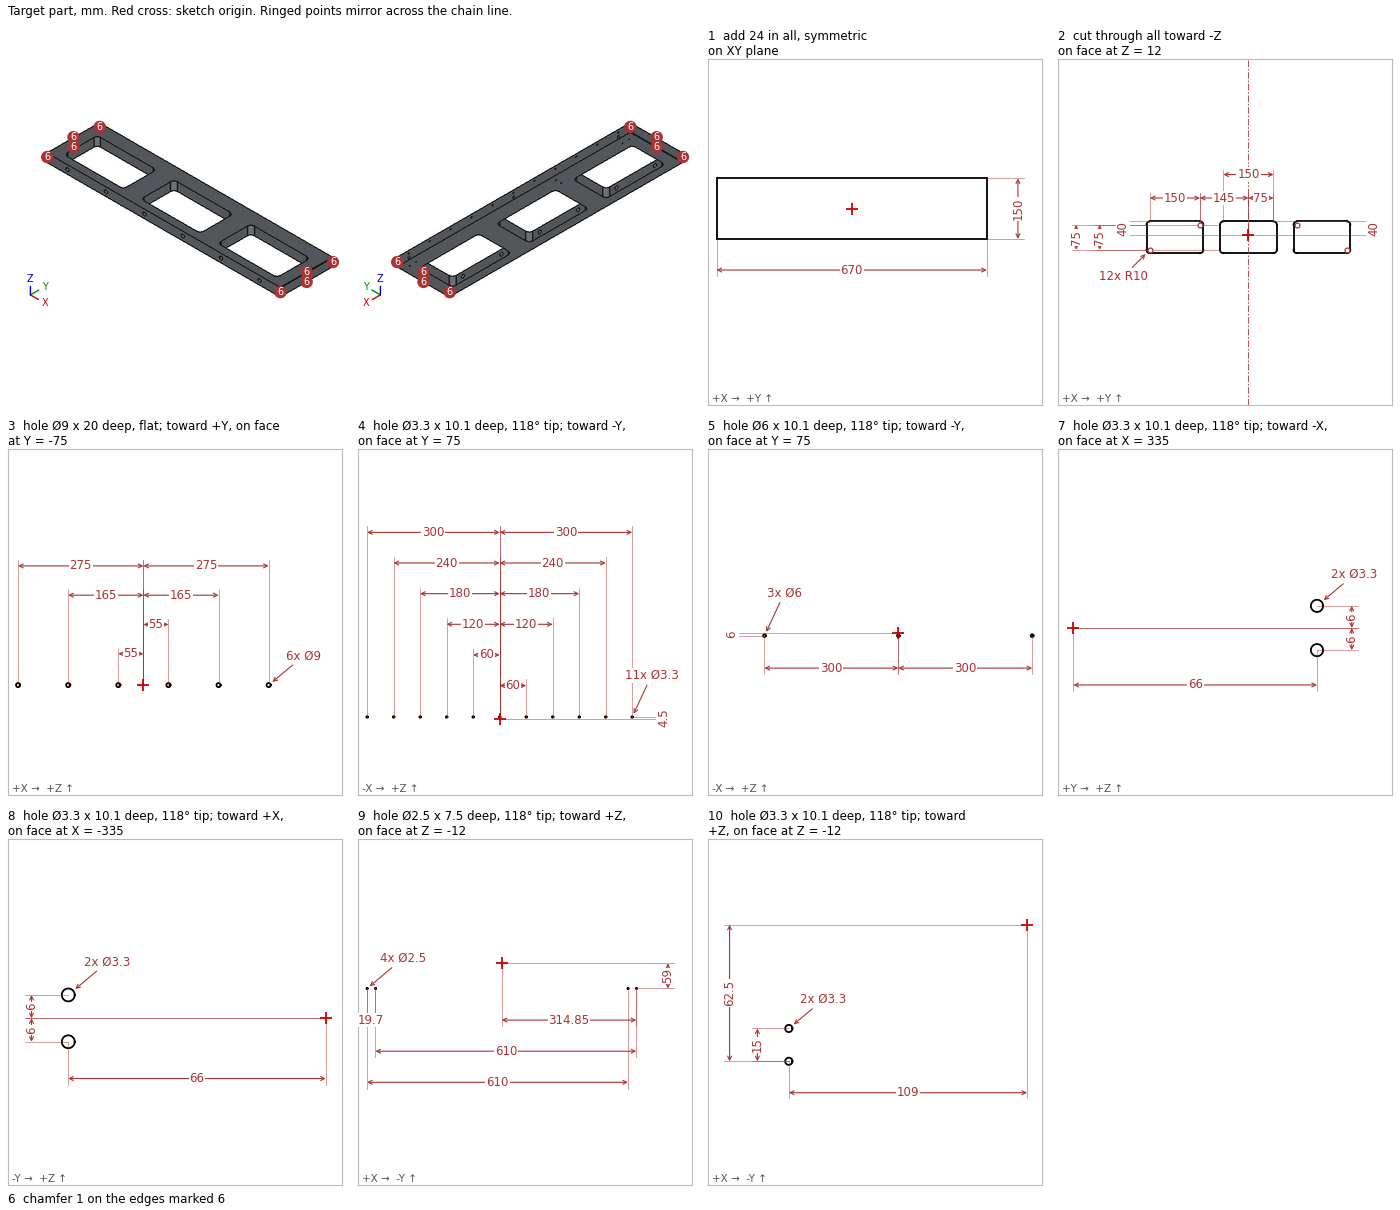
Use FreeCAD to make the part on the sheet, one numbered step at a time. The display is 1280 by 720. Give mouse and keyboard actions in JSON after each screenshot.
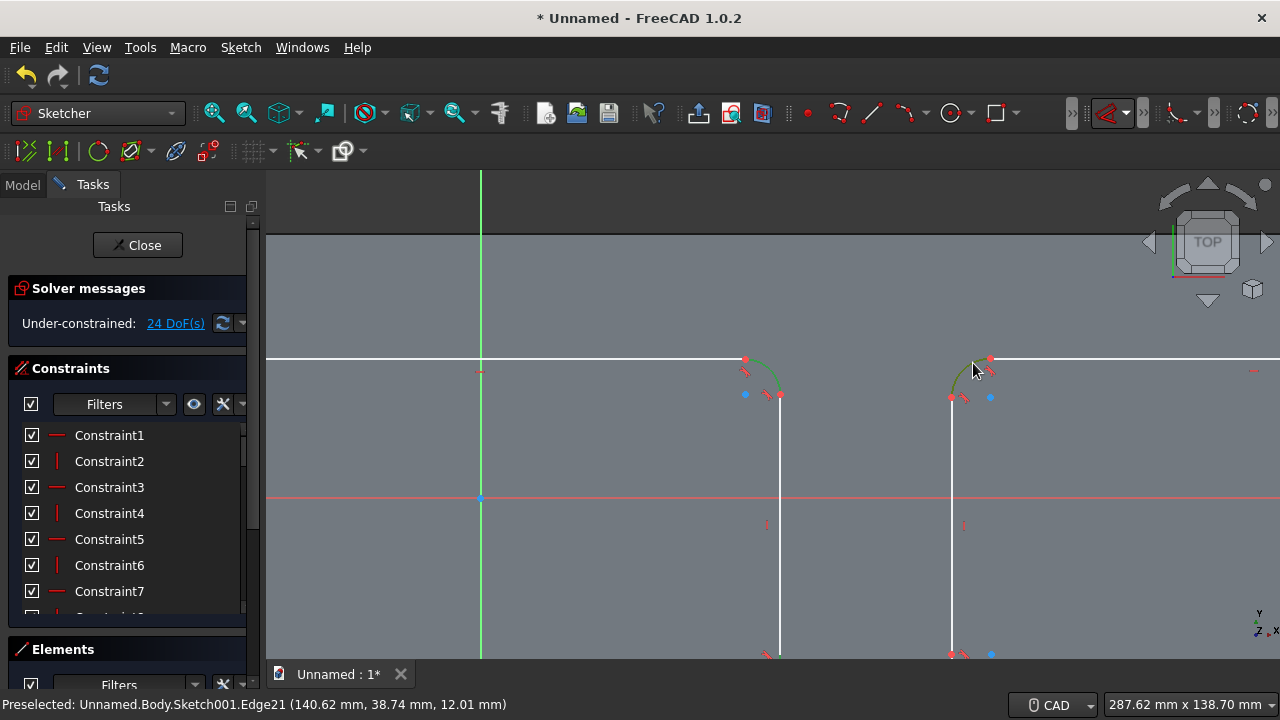
{"action": "scroll", "coordinate": [778, 378], "scroll_direction": "down", "scroll_amount": 7}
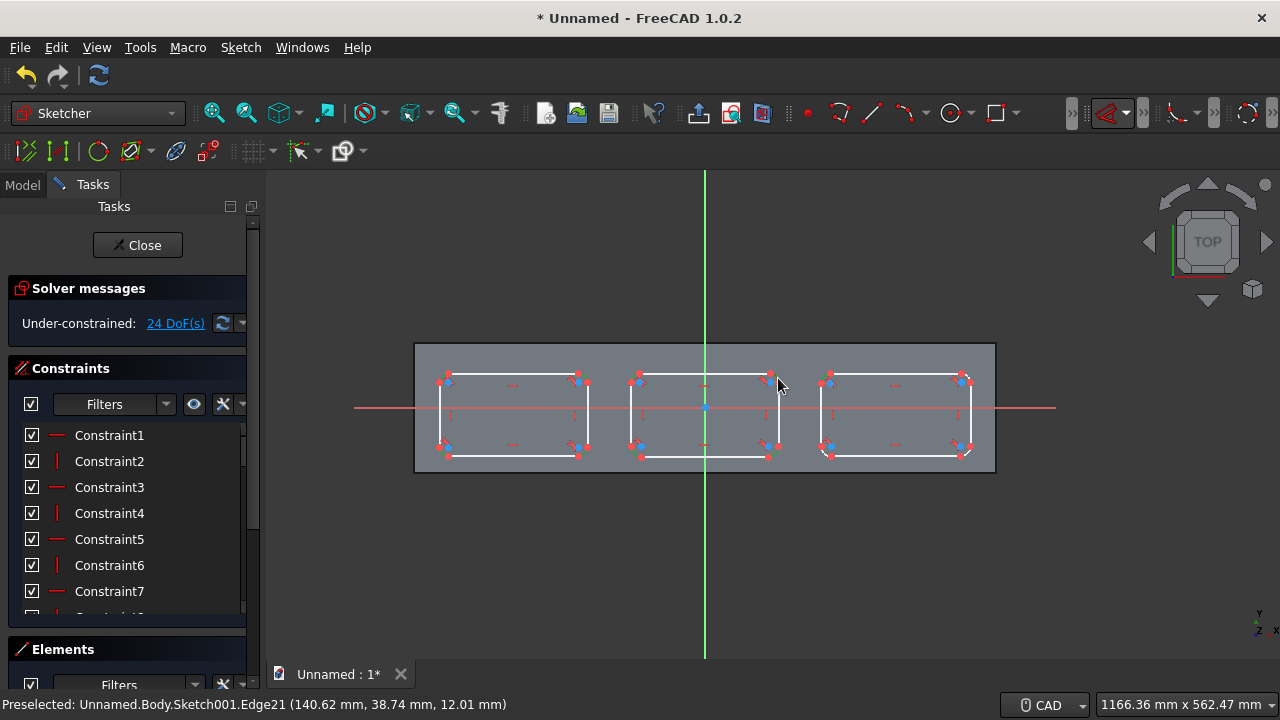
{"action": "scroll", "coordinate": [822, 451], "scroll_direction": "up", "scroll_amount": 6}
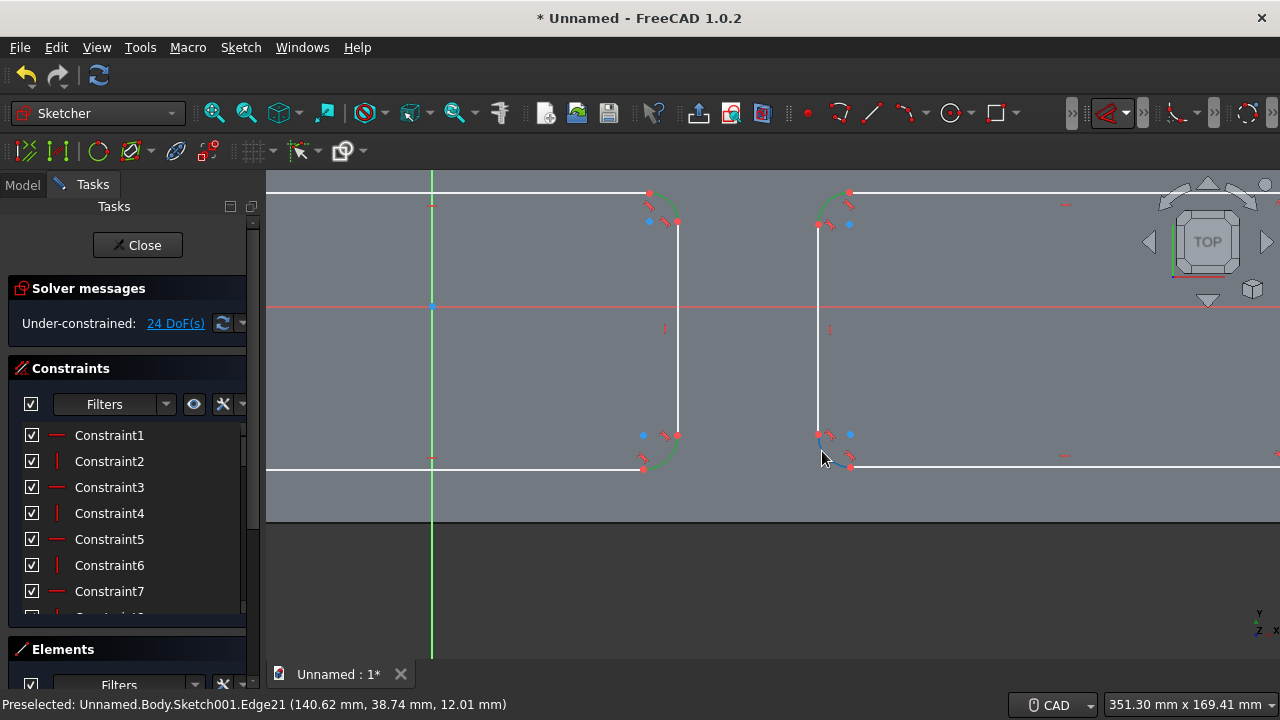
{"action": "left_click", "coordinate": [822, 450]}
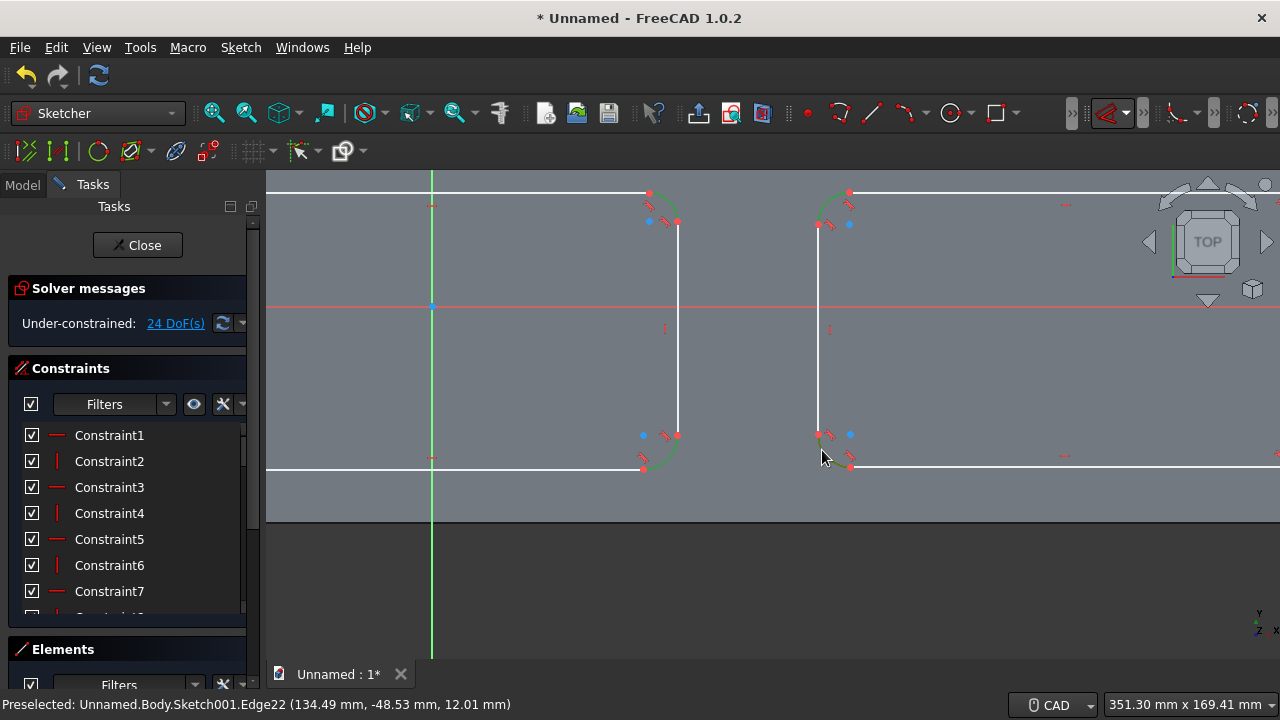
{"action": "scroll", "coordinate": [822, 452], "scroll_direction": "down", "scroll_amount": 6}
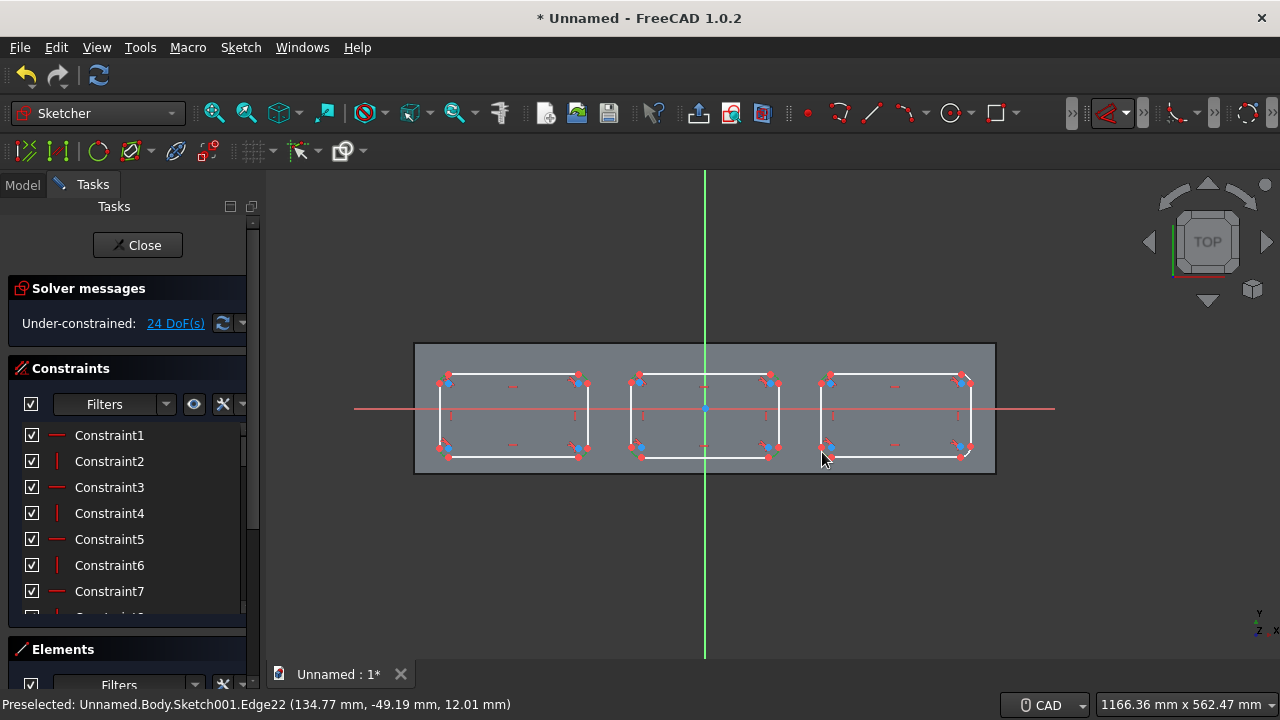
{"action": "scroll", "coordinate": [965, 456], "scroll_direction": "up", "scroll_amount": 6}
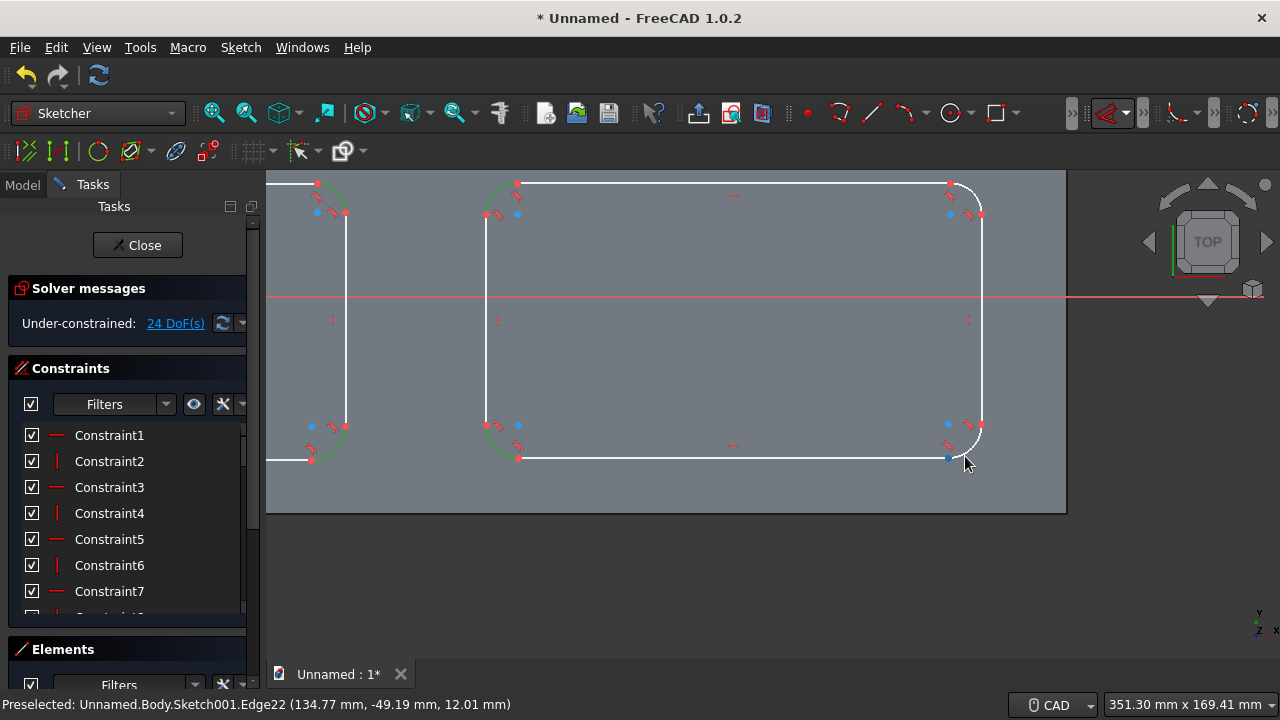
{"action": "left_click", "coordinate": [963, 454]}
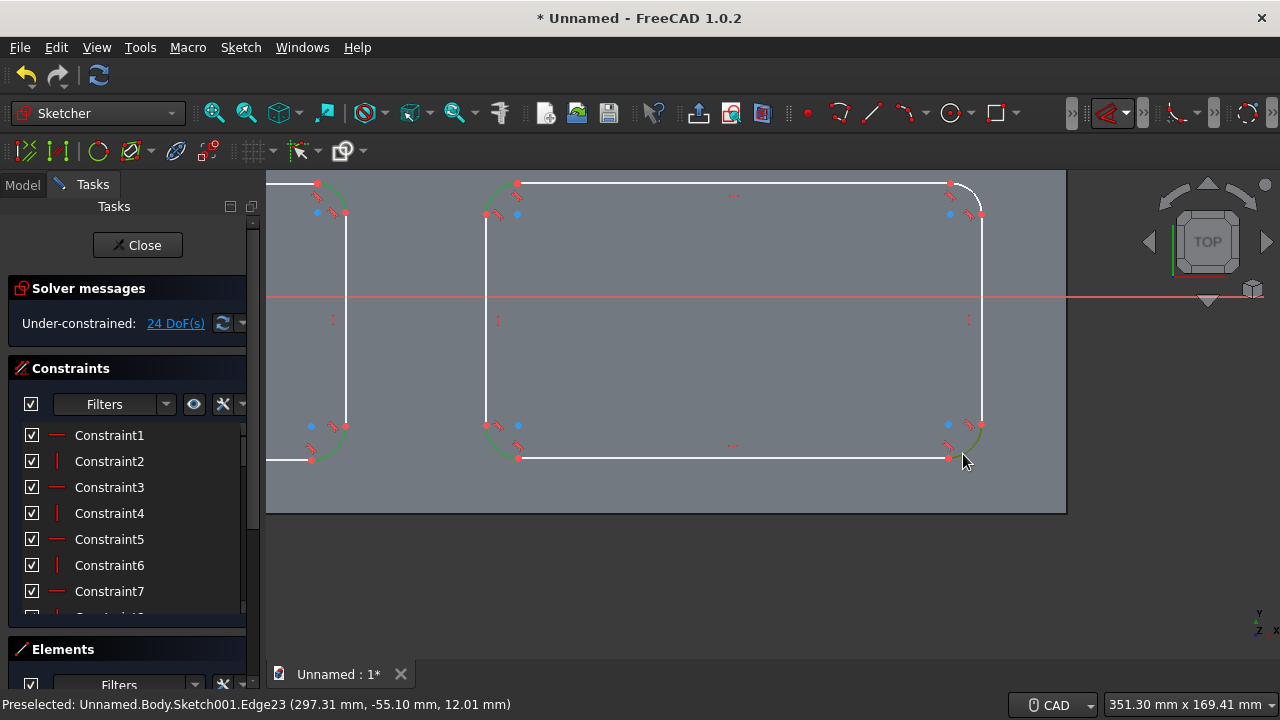
{"action": "left_click", "coordinate": [978, 200]}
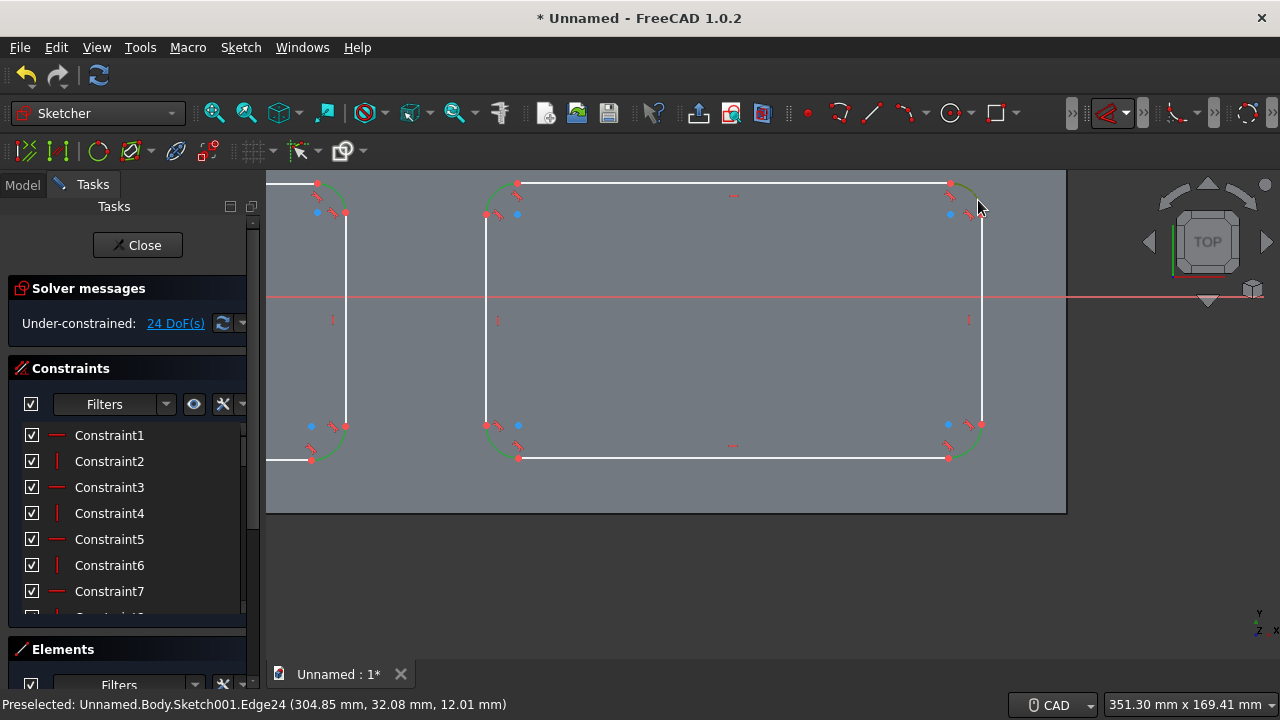
{"action": "key", "text": "e"}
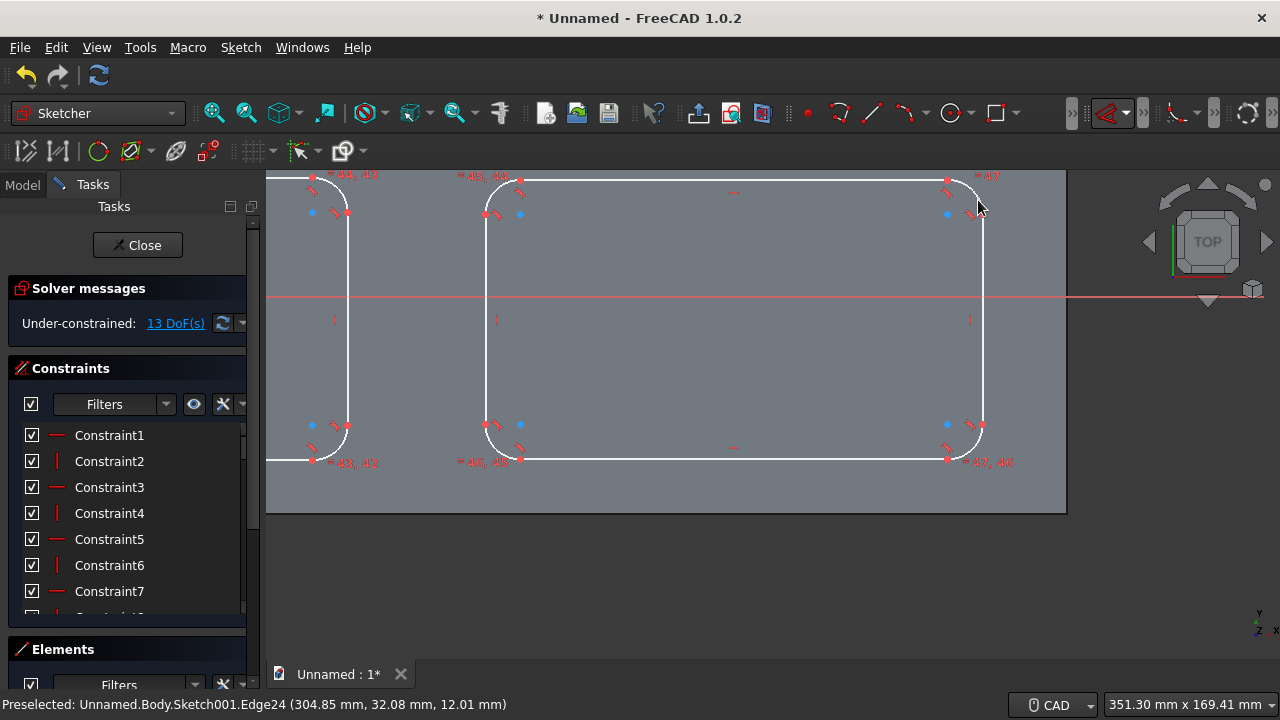
{"action": "scroll", "coordinate": [965, 456], "scroll_direction": "down", "scroll_amount": 6}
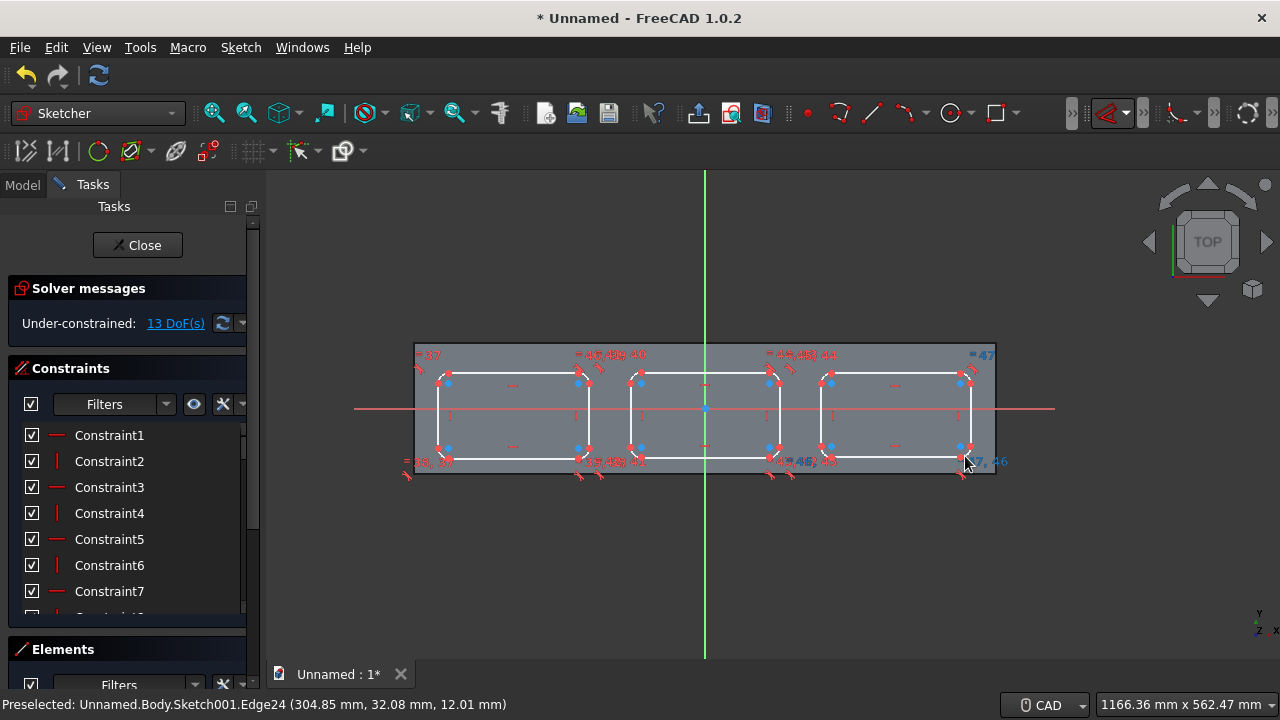
{"action": "left_click", "coordinate": [579, 384]}